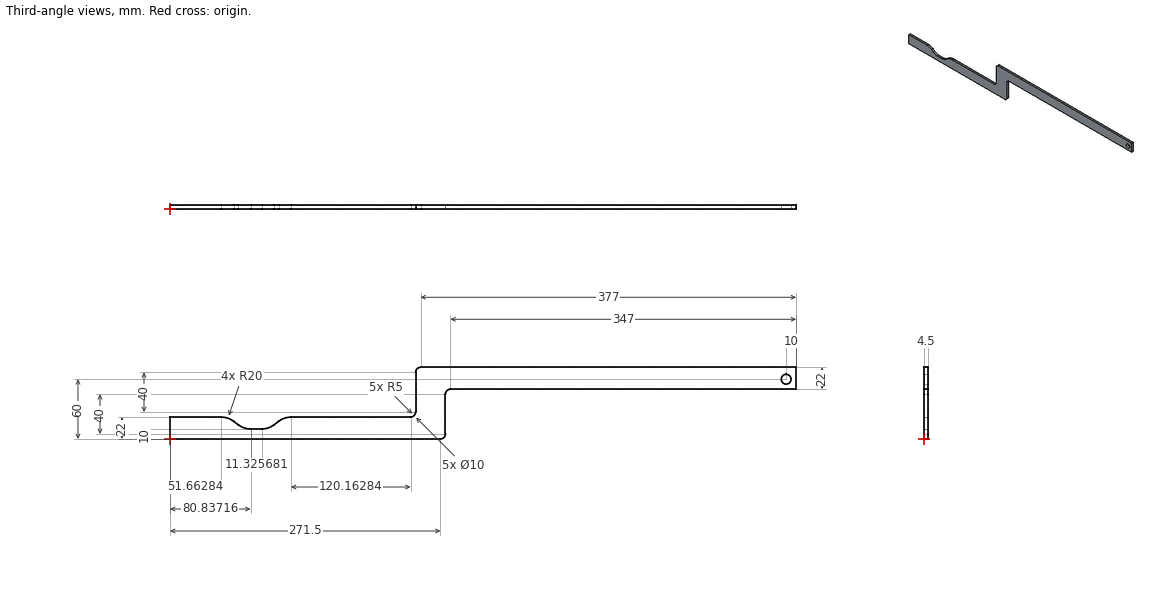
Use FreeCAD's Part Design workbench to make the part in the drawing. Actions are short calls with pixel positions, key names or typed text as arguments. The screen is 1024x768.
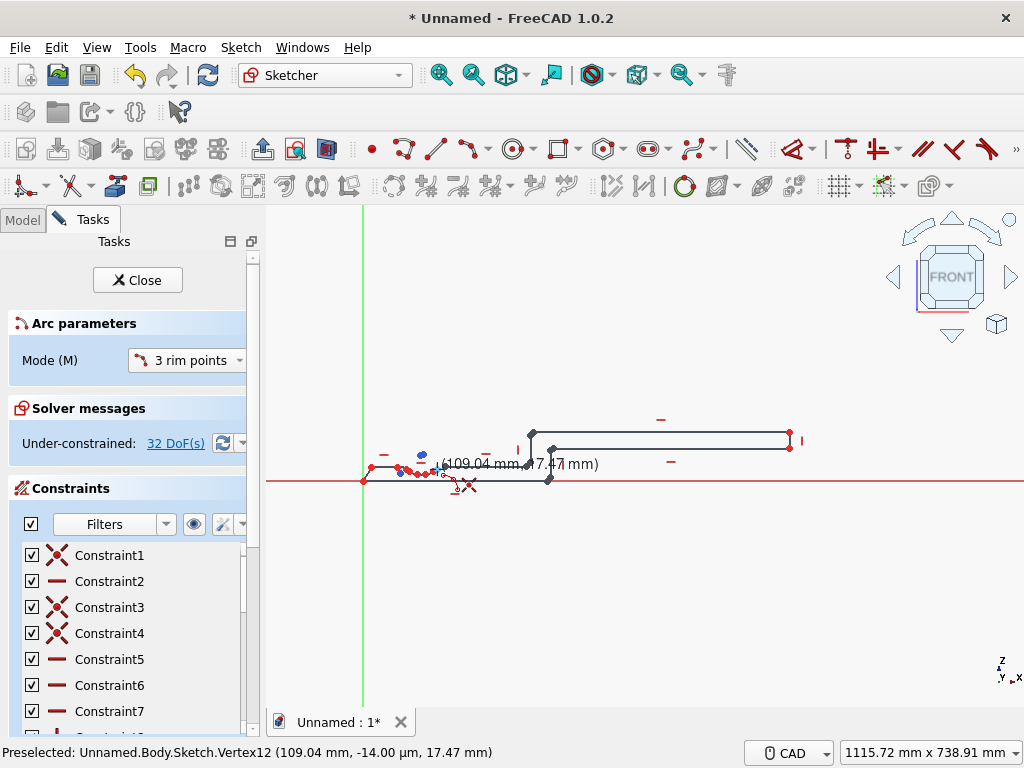
scroll(446, 466, up, 3)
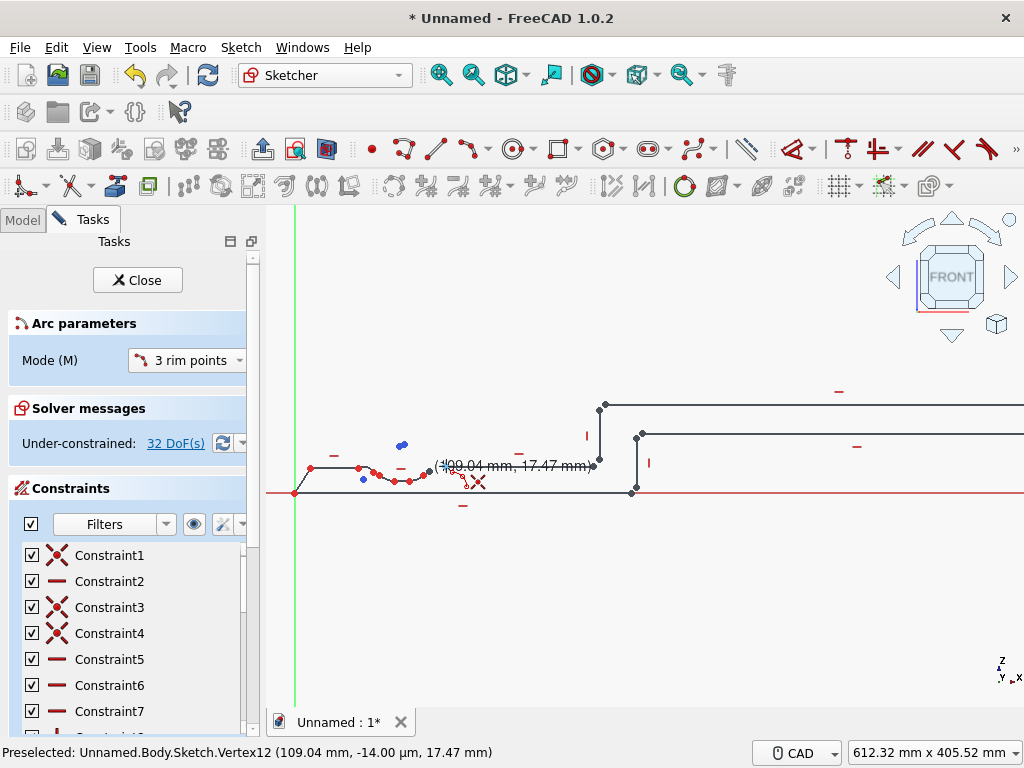
click(445, 467)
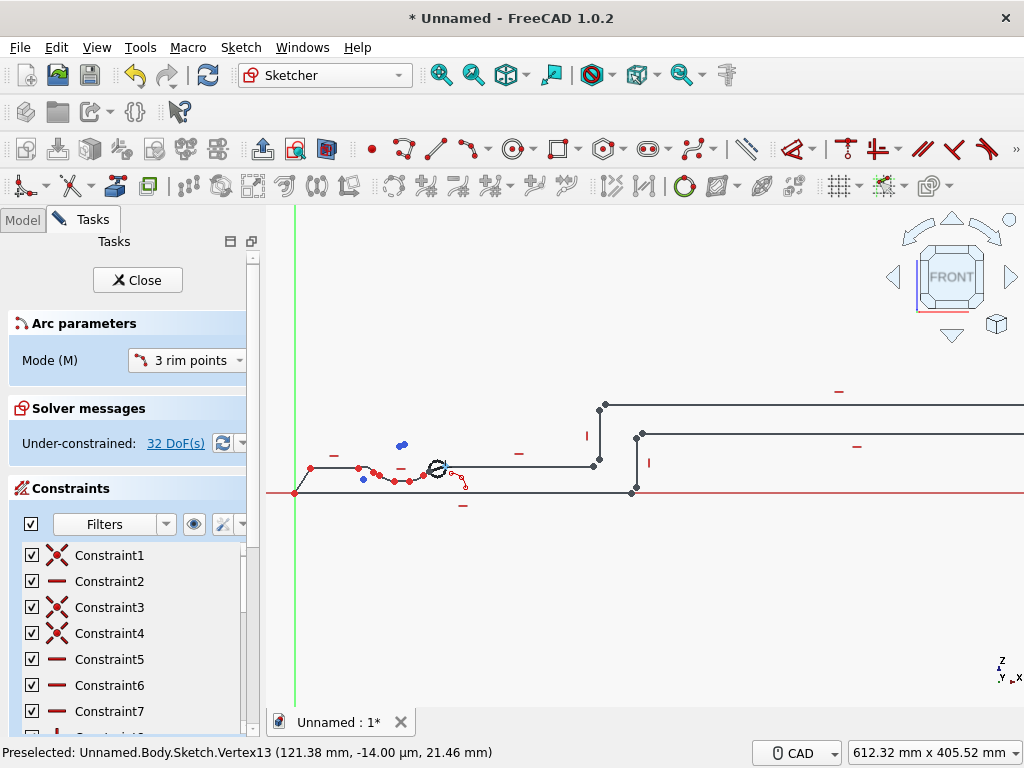
scroll(437, 467, up, 13)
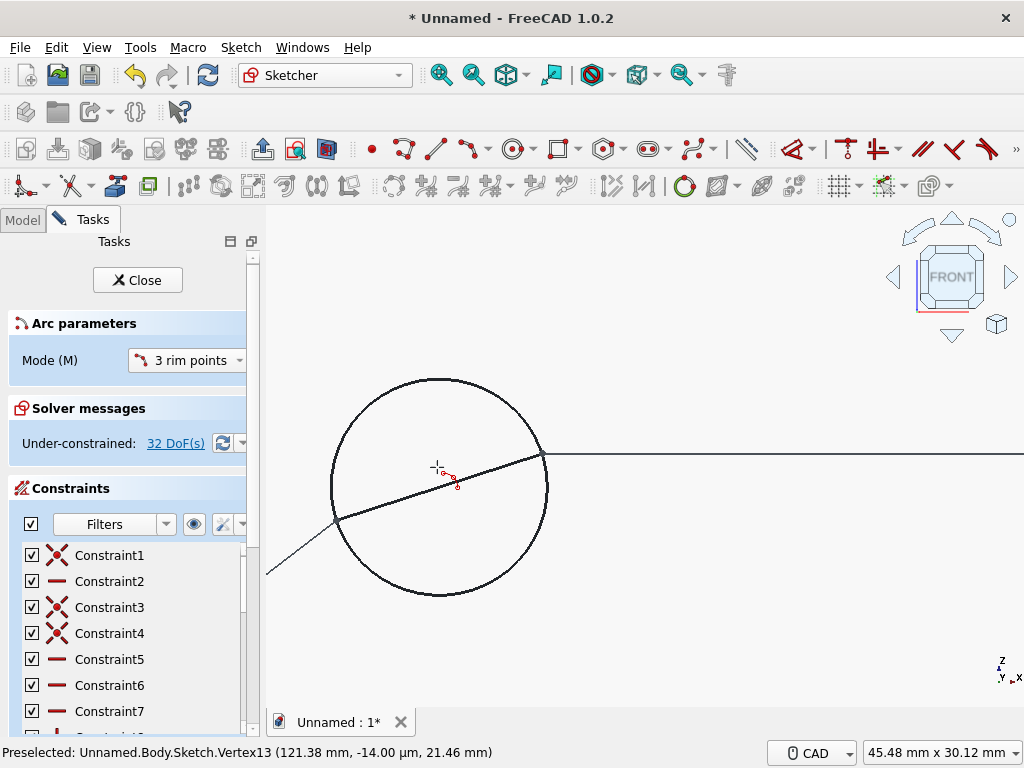
click(434, 463)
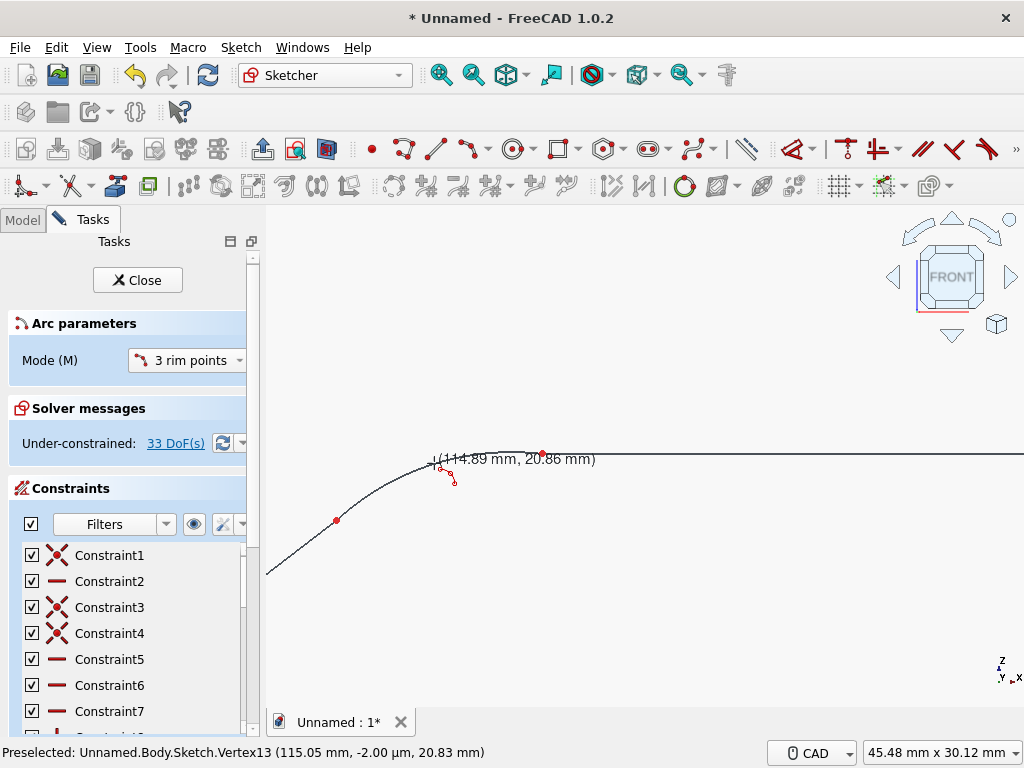
scroll(441, 466, down, 16)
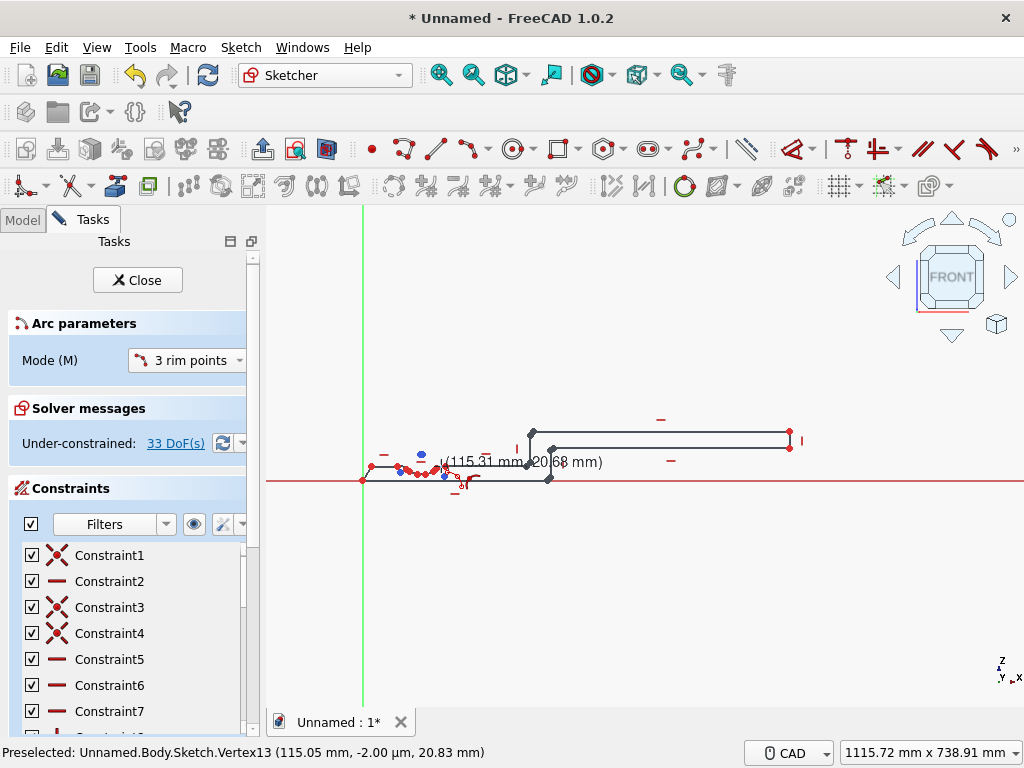
scroll(527, 466, up, 6)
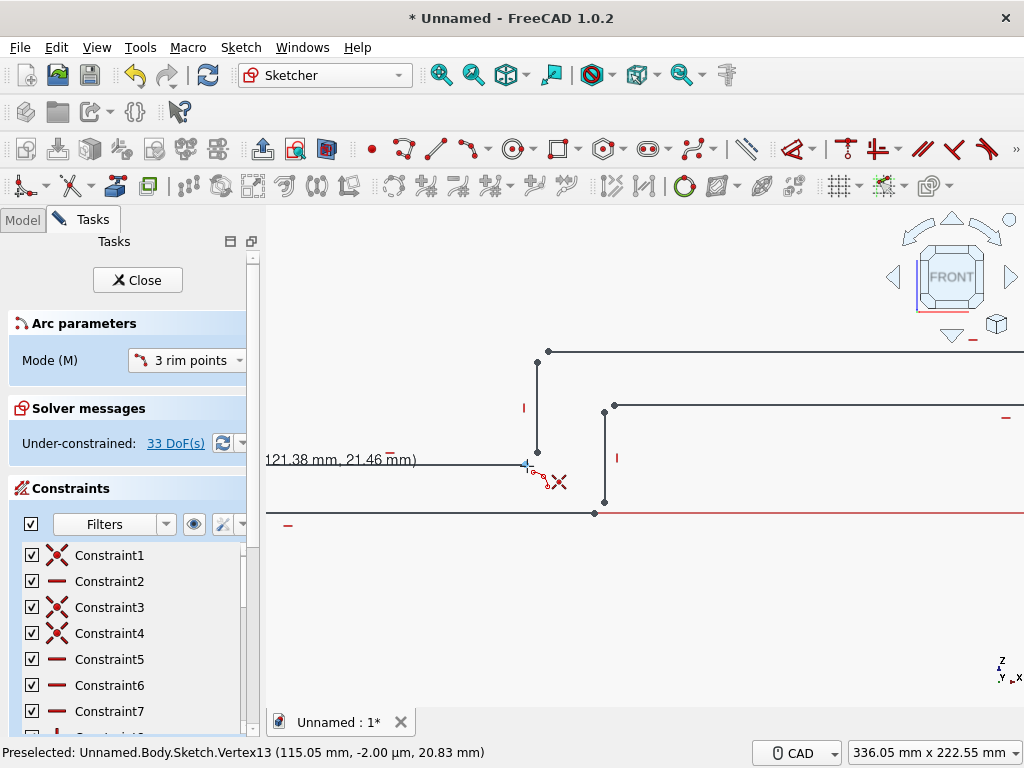
click(525, 465)
click(537, 453)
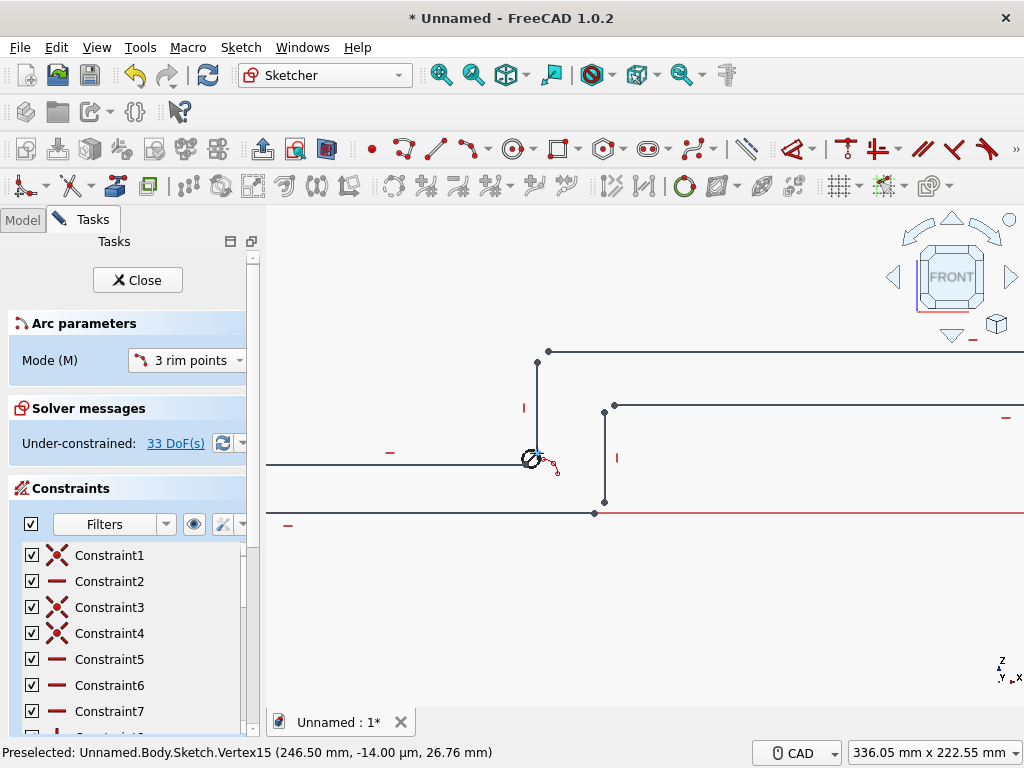
scroll(534, 460, up, 8)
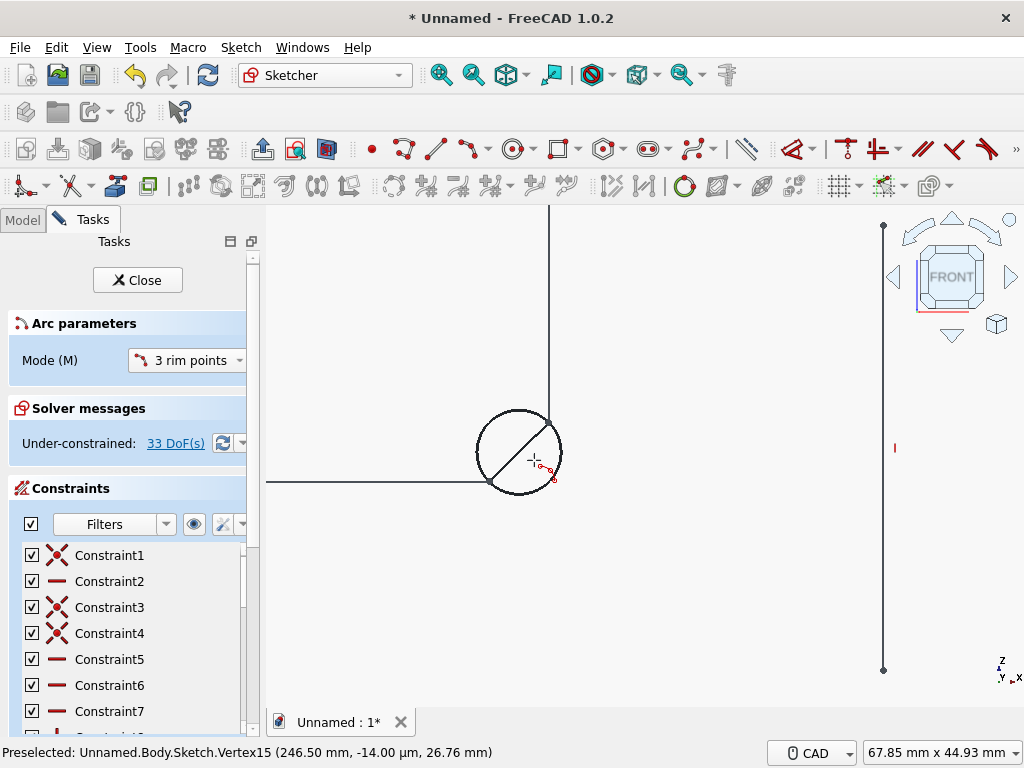
click(533, 459)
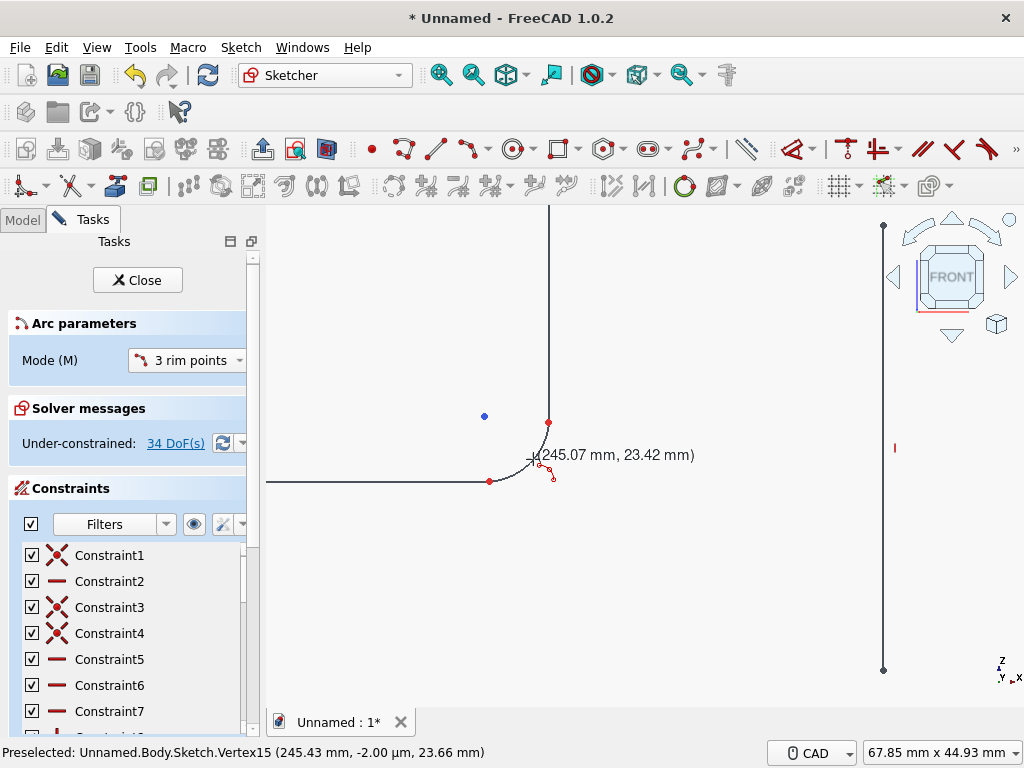
scroll(529, 465, down, 14)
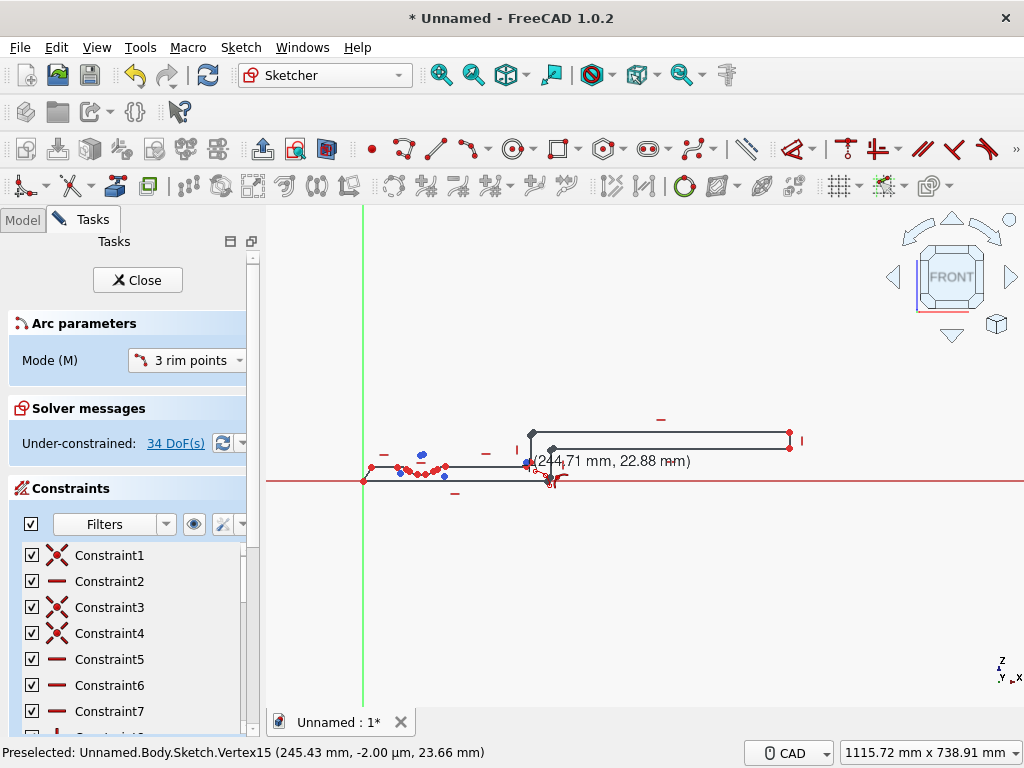
scroll(531, 436, up, 6)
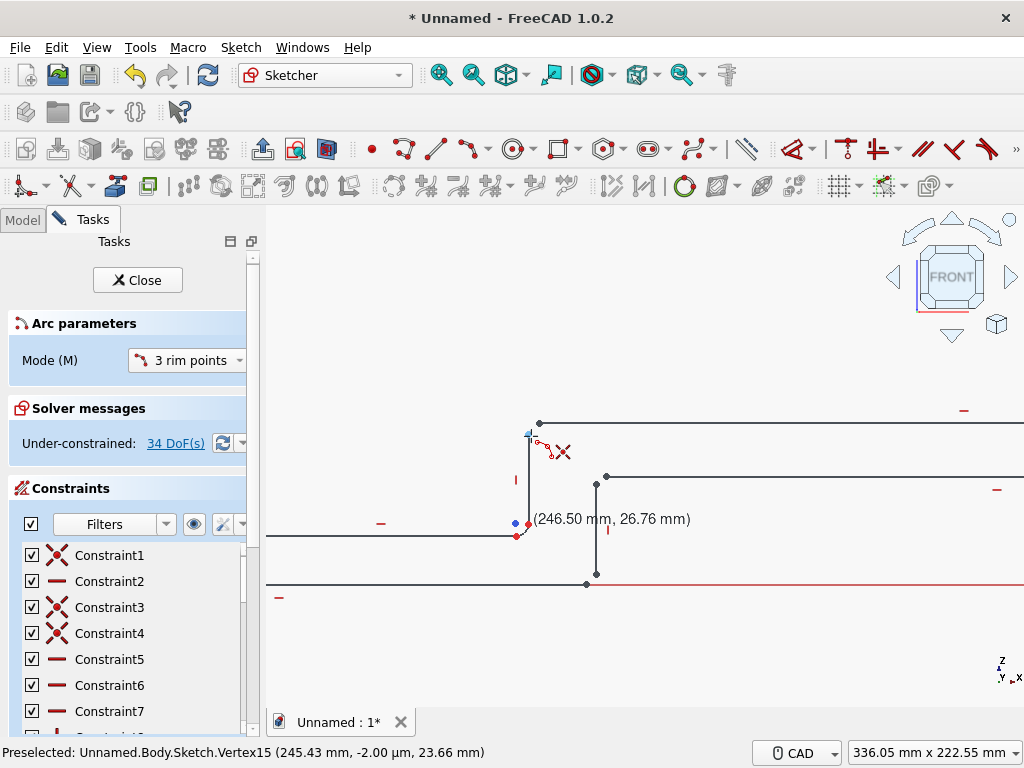
click(529, 434)
click(540, 423)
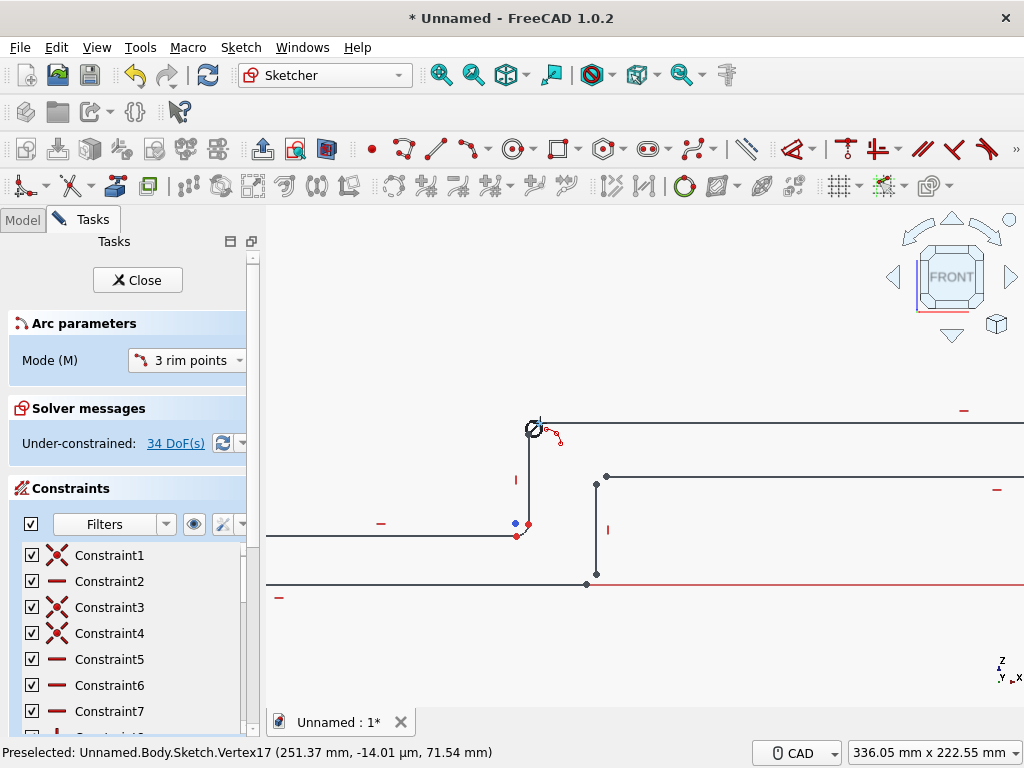
scroll(532, 426, up, 8)